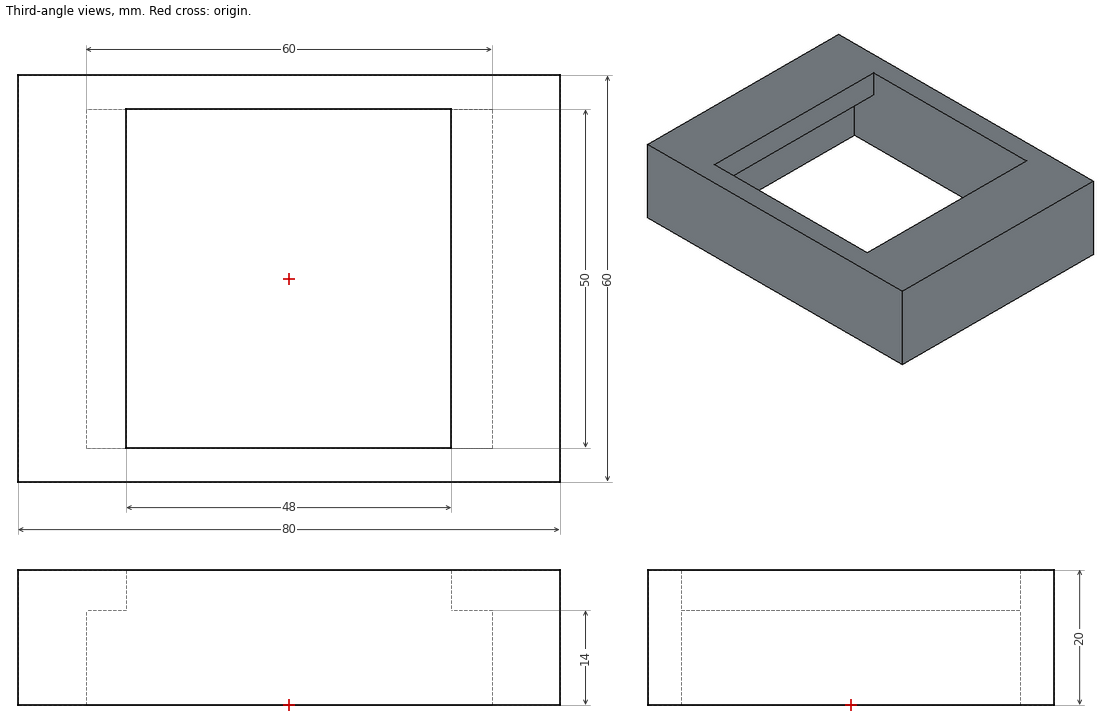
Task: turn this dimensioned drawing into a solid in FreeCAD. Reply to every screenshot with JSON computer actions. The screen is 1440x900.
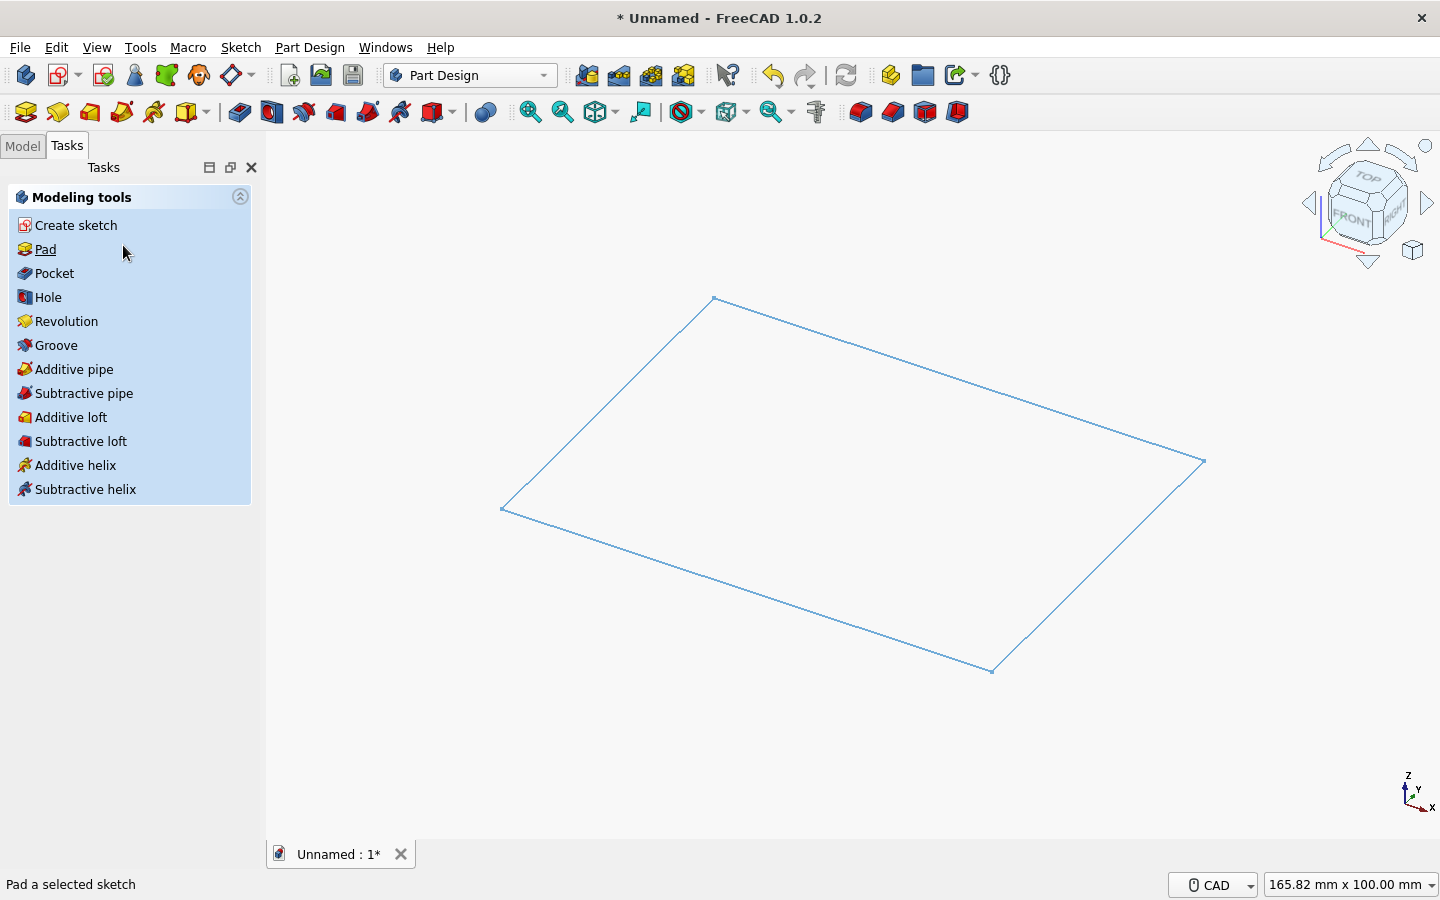
{"action": "left_click", "coordinate": [26, 112]}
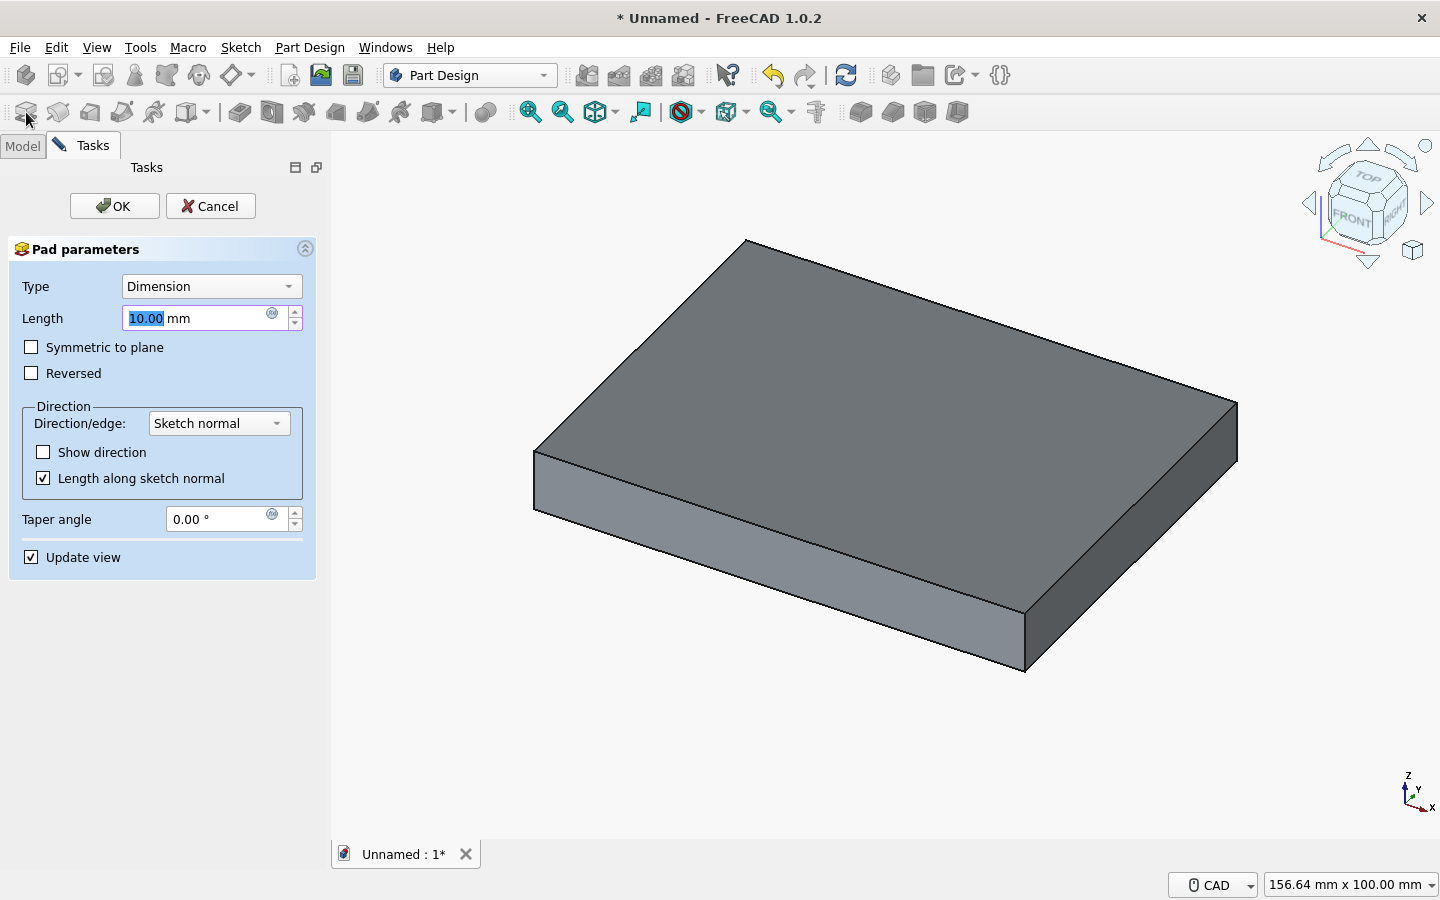
{"action": "type", "text": "20"}
{"action": "key", "text": "Tab"}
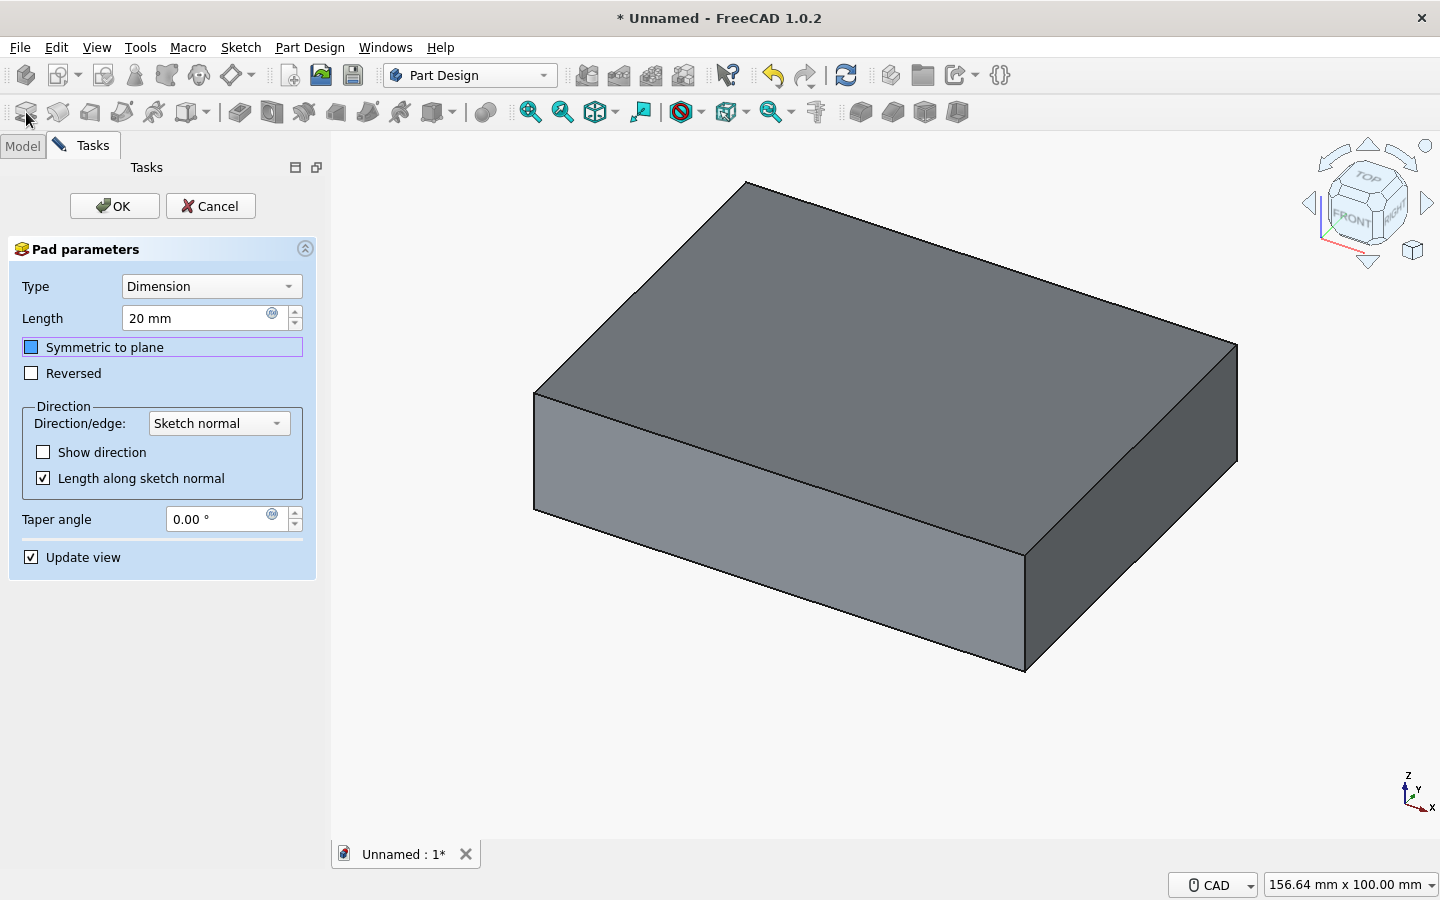
{"action": "left_click", "coordinate": [115, 206]}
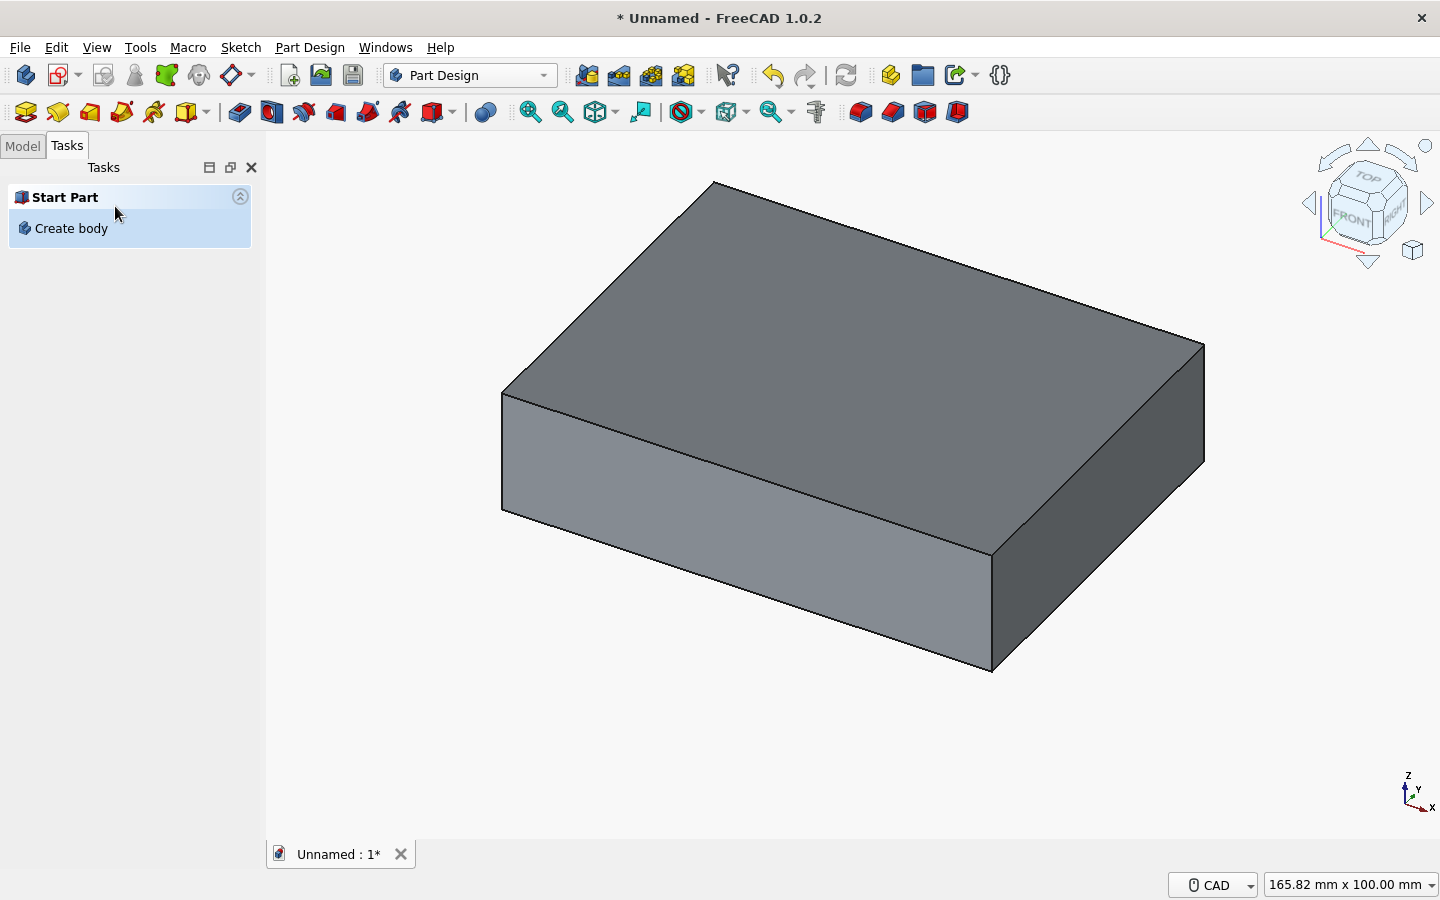
{"action": "left_click", "coordinate": [853, 368]}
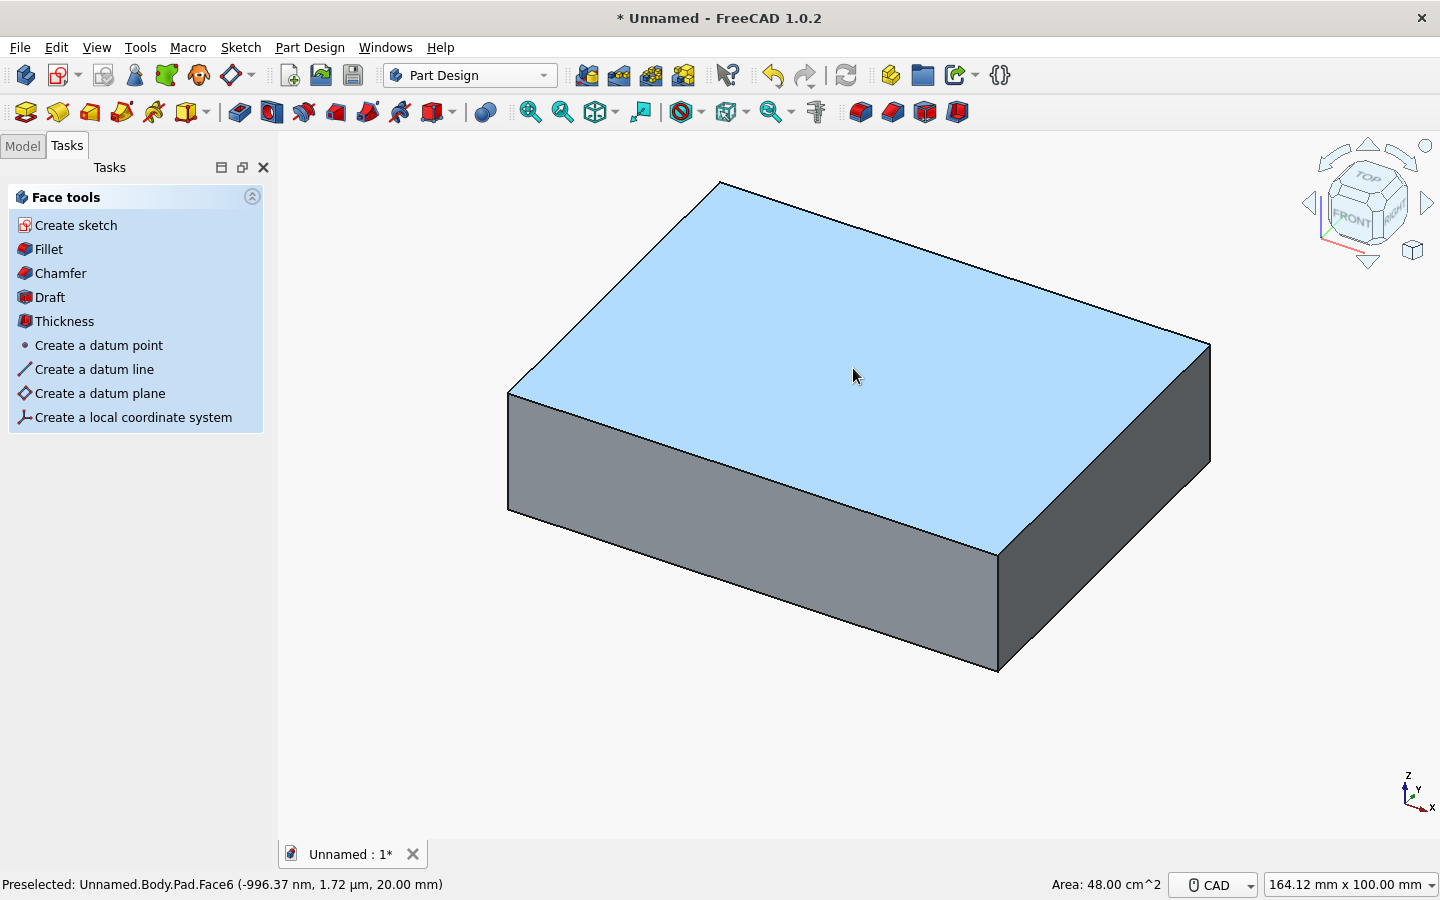
{"action": "left_click", "coordinate": [58, 76]}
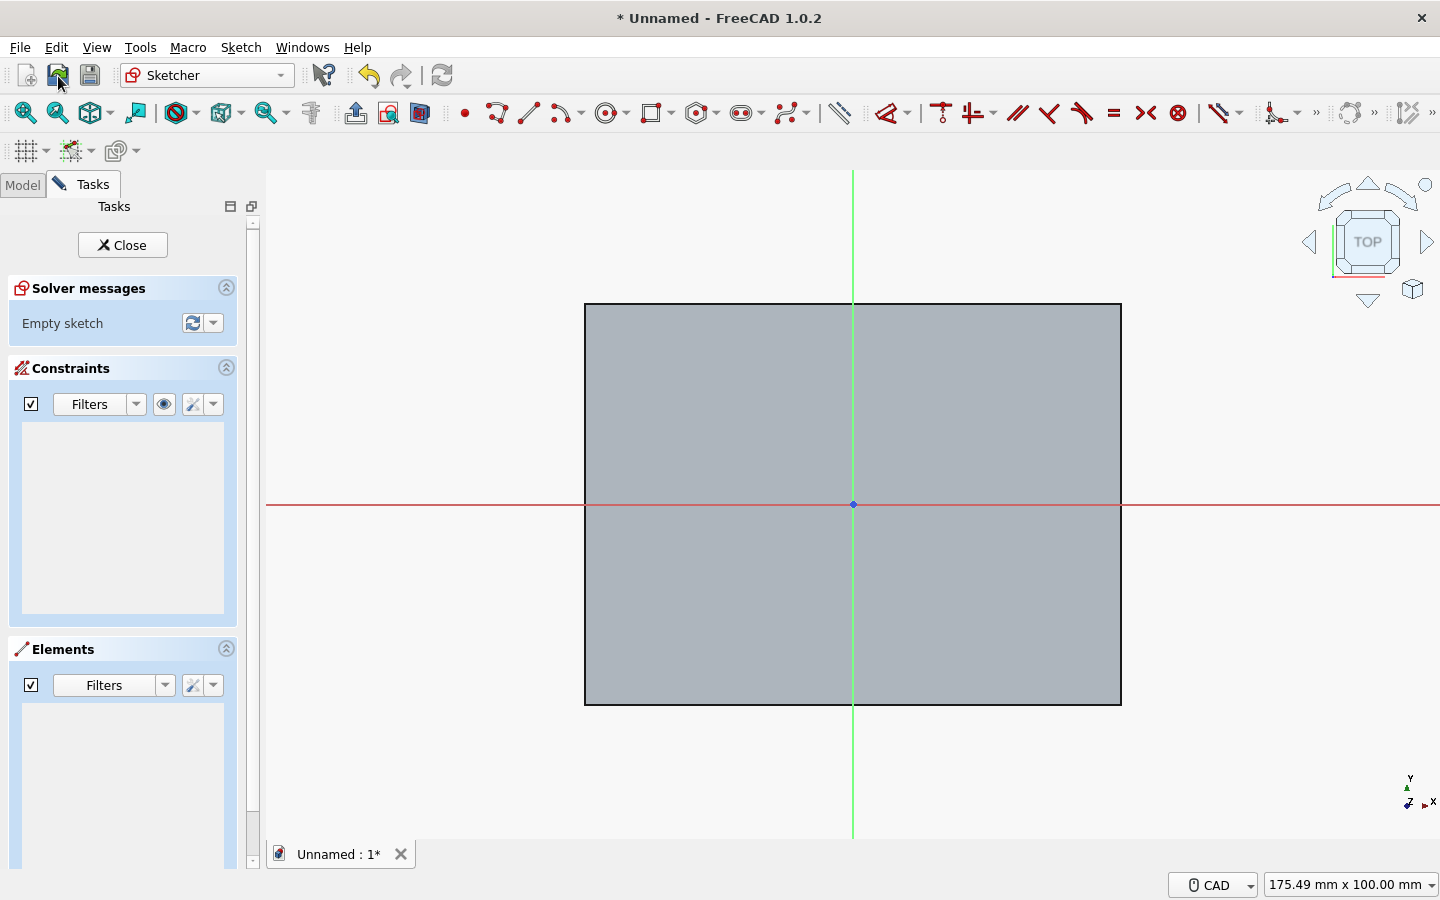
{"action": "key", "text": "g v"}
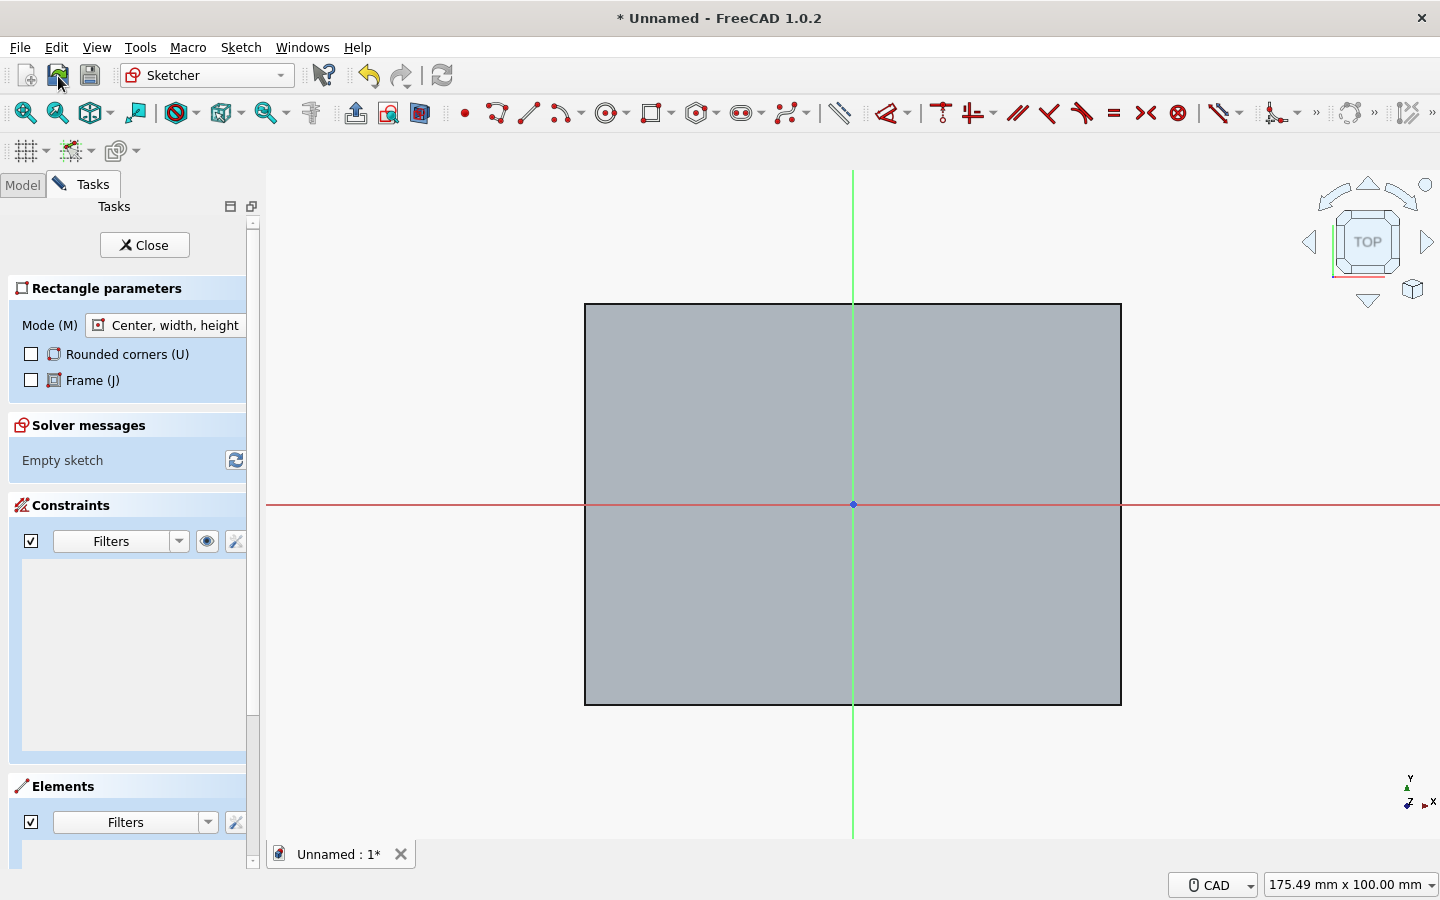
{"action": "left_click", "coordinate": [853, 504]}
{"action": "mouse_move", "coordinate": [1014, 337]}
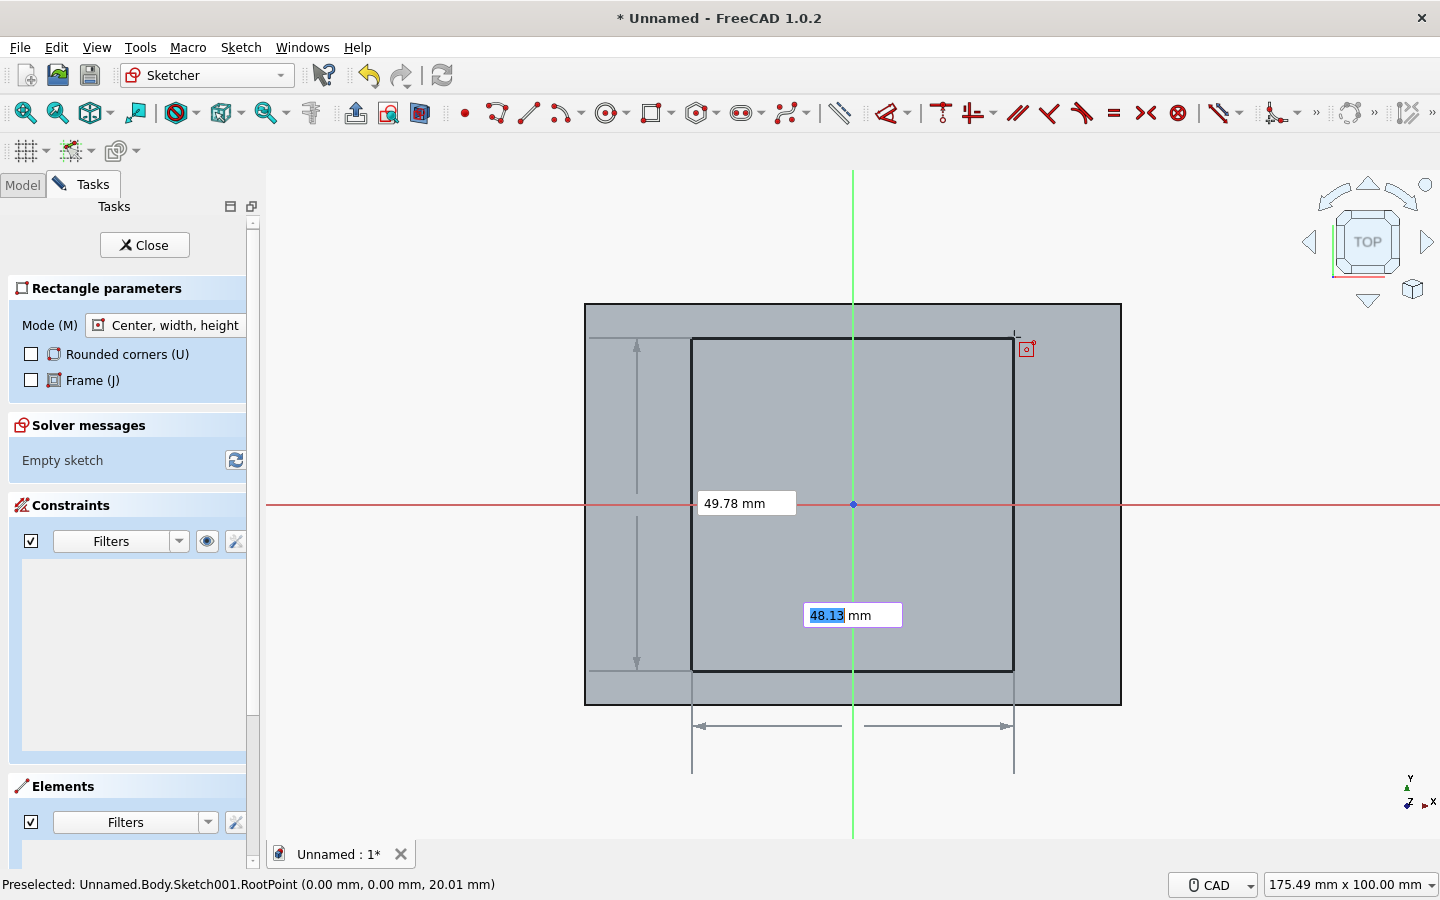
{"action": "type", "text": "48"}
{"action": "key", "text": "Tab"}
{"action": "type", "text": "50"}
{"action": "key", "text": "Return"}
{"action": "key", "text": "Escape"}